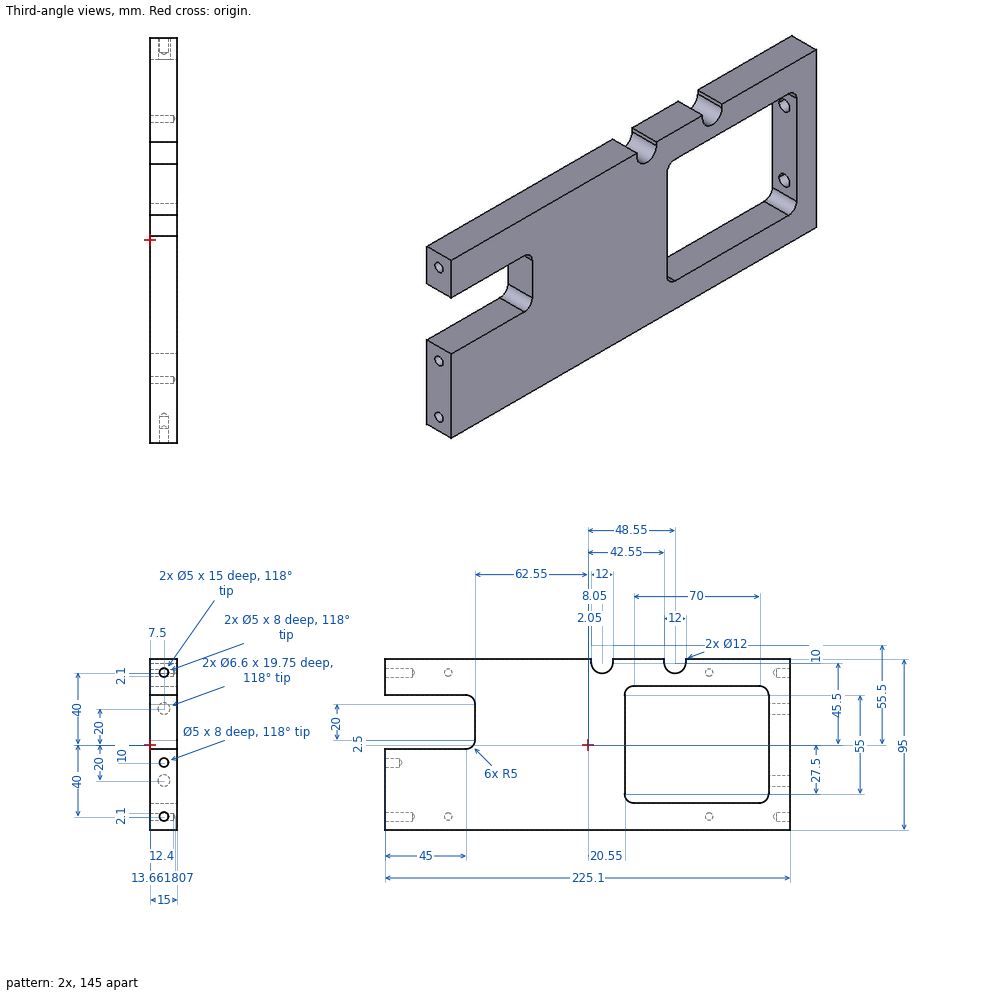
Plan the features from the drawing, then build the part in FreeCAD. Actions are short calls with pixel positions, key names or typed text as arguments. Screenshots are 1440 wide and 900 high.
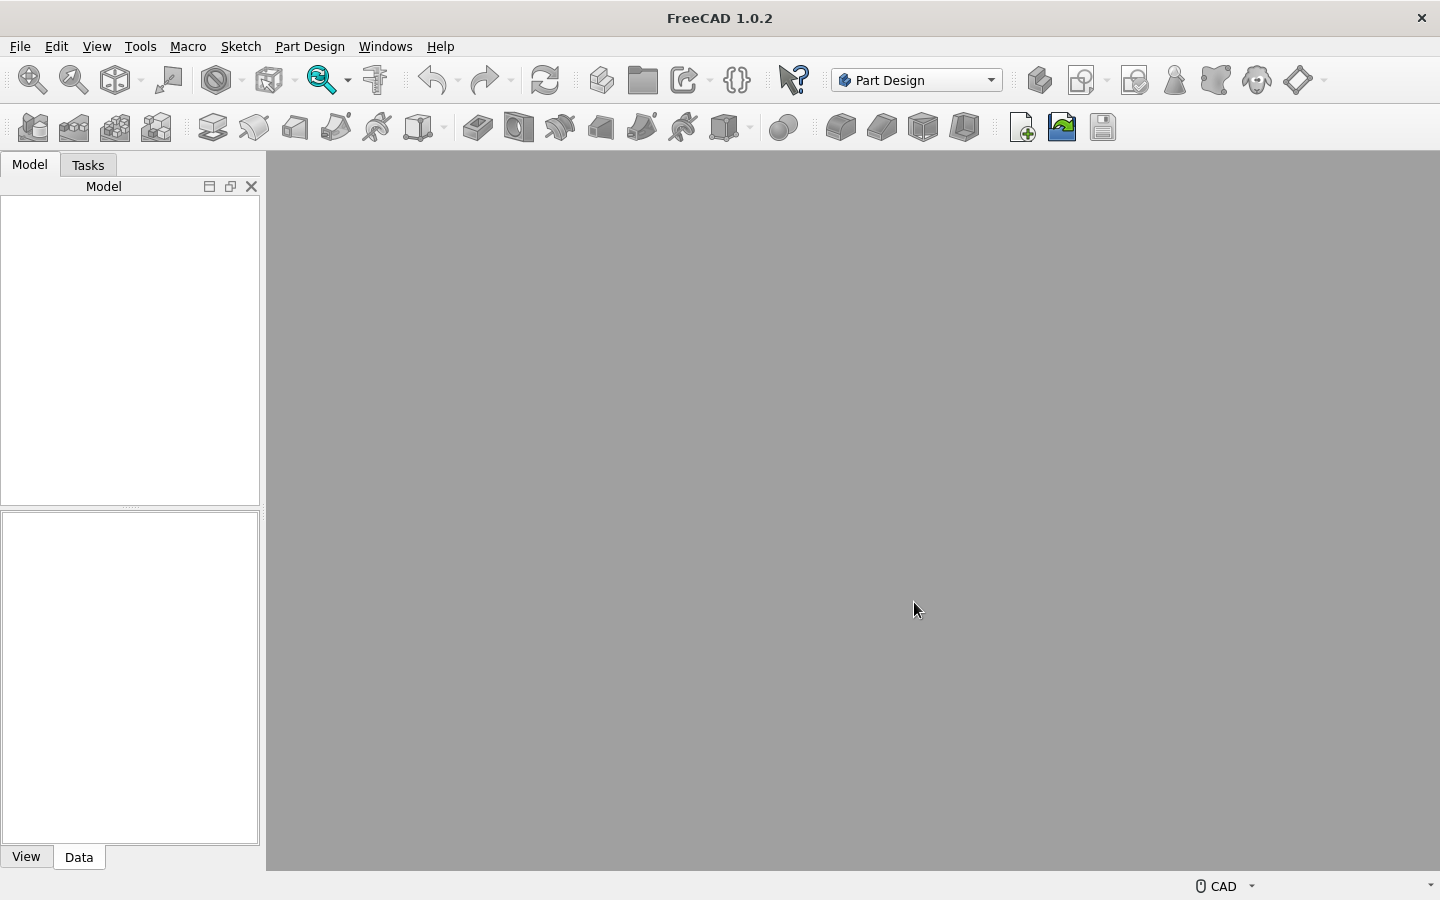
click(1021, 128)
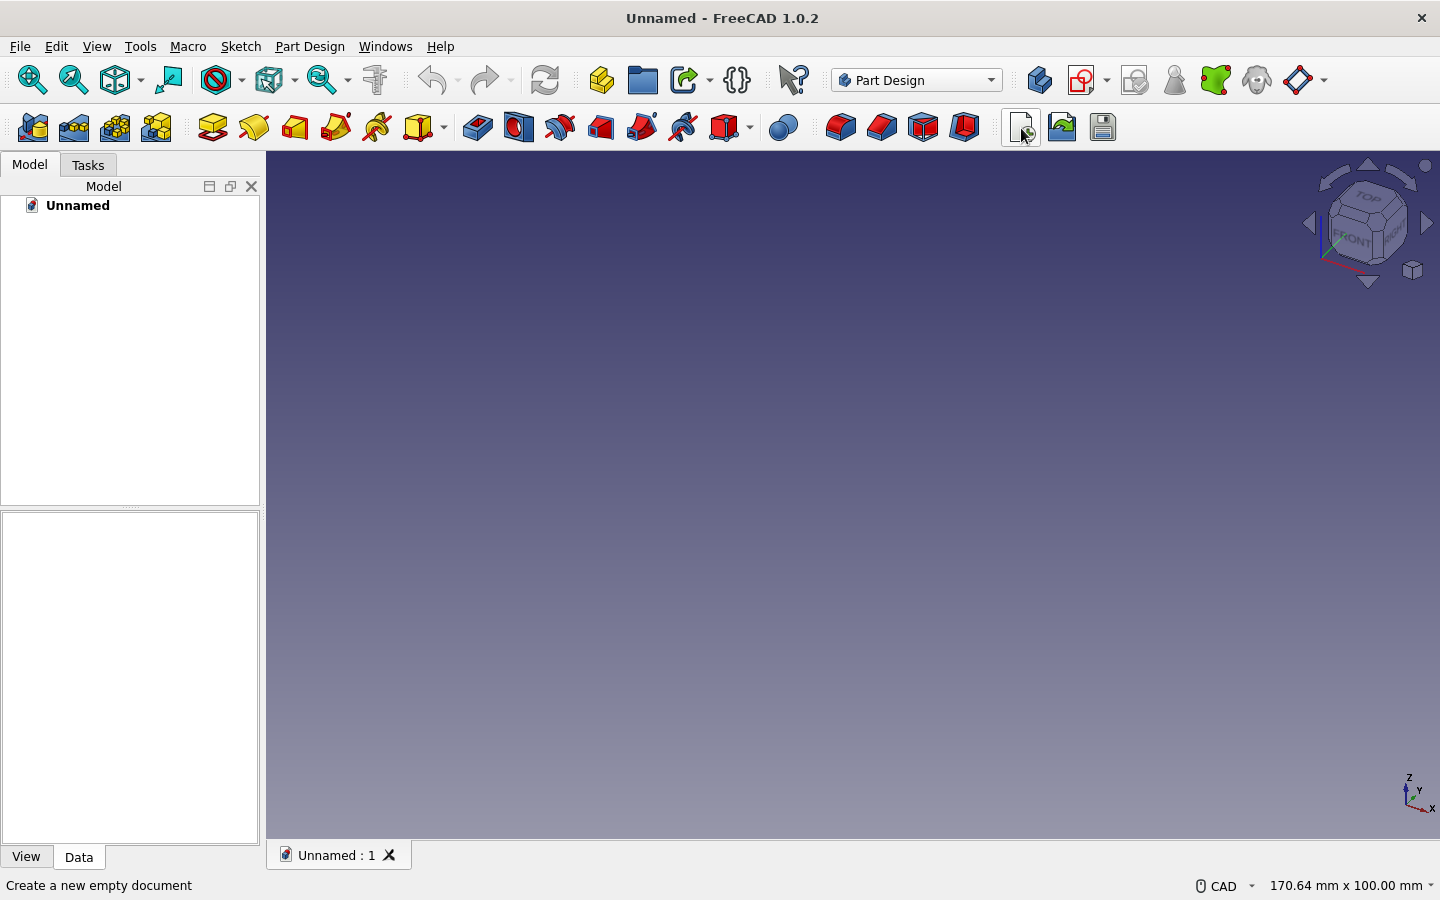
click(1080, 80)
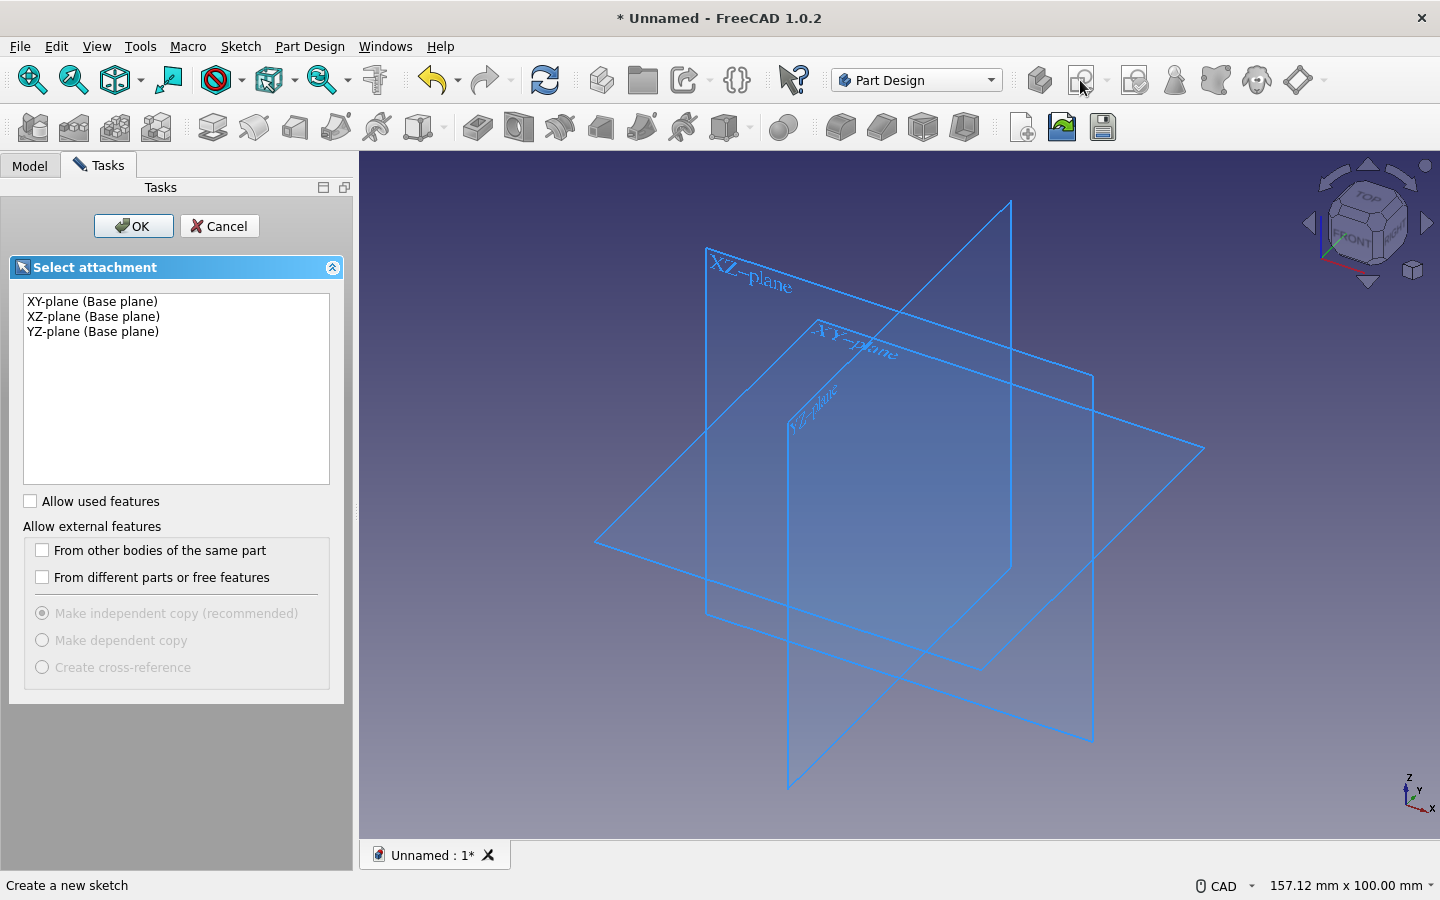
click(84, 332)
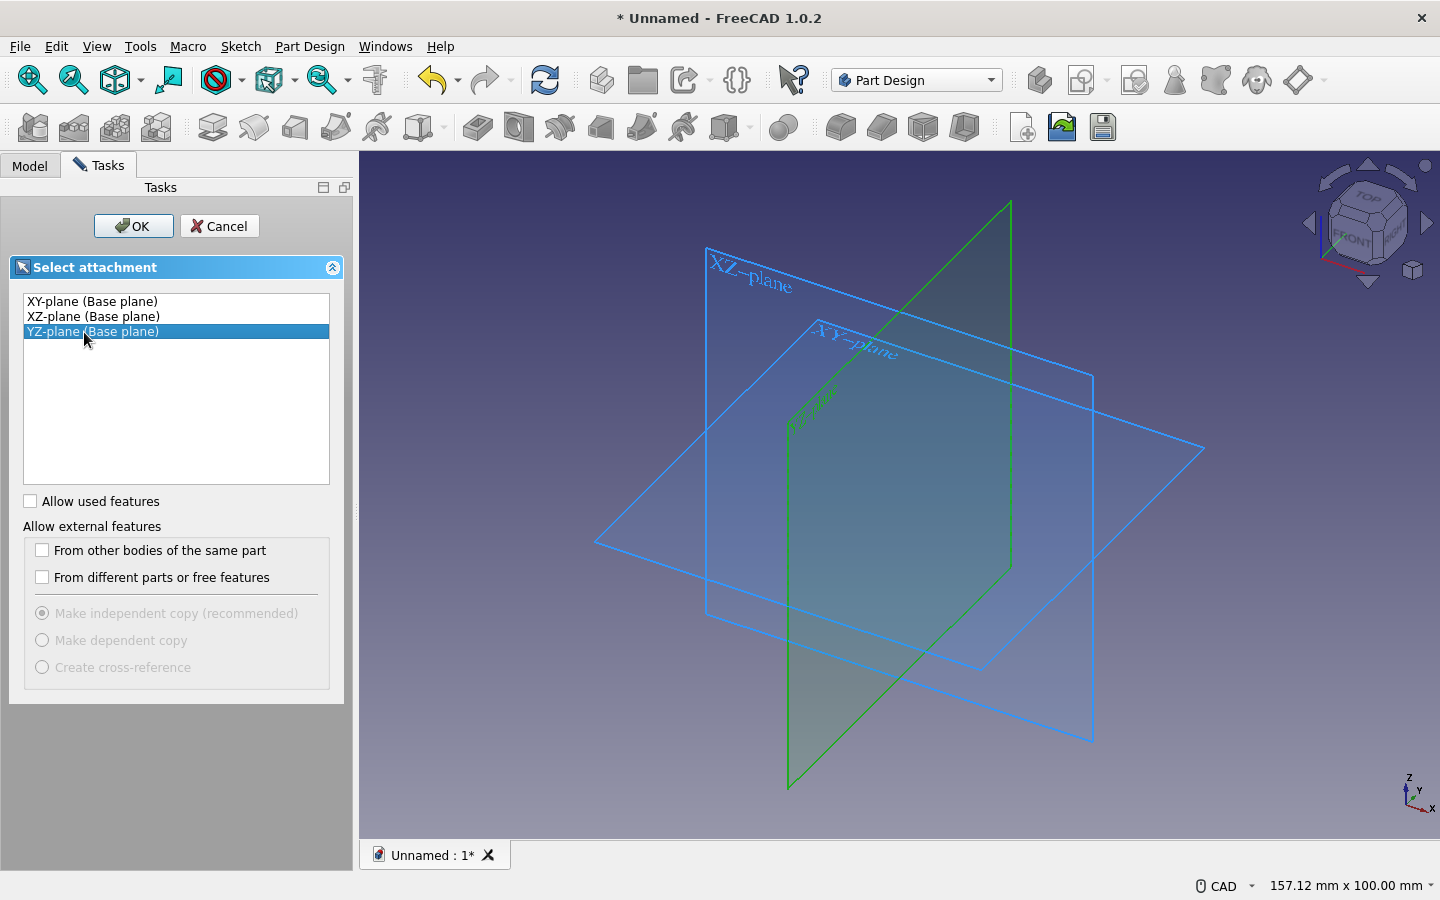
click(134, 226)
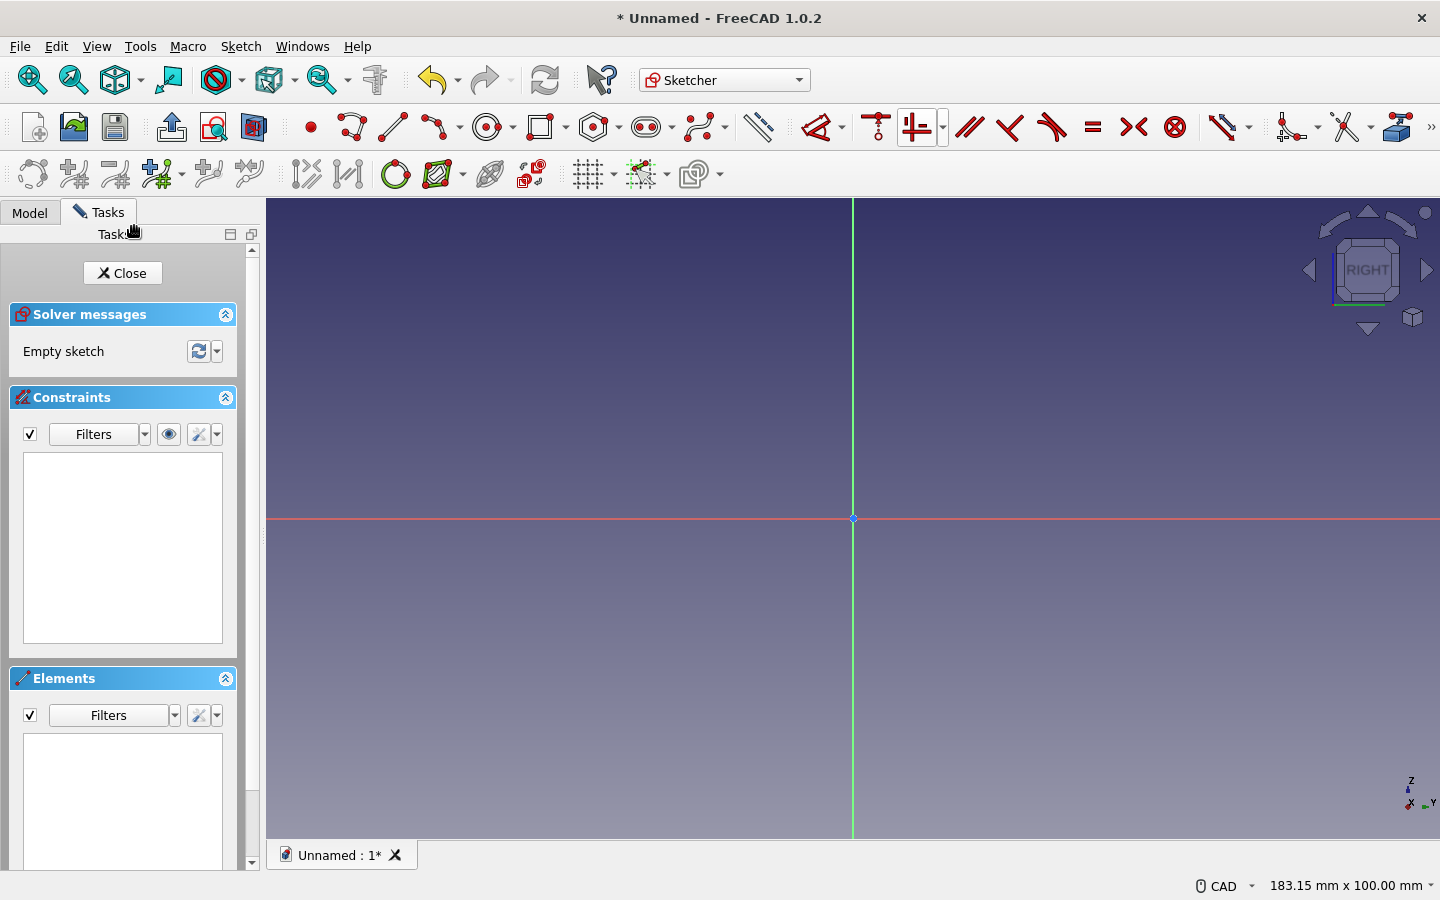
scroll(729, 519, down, 4)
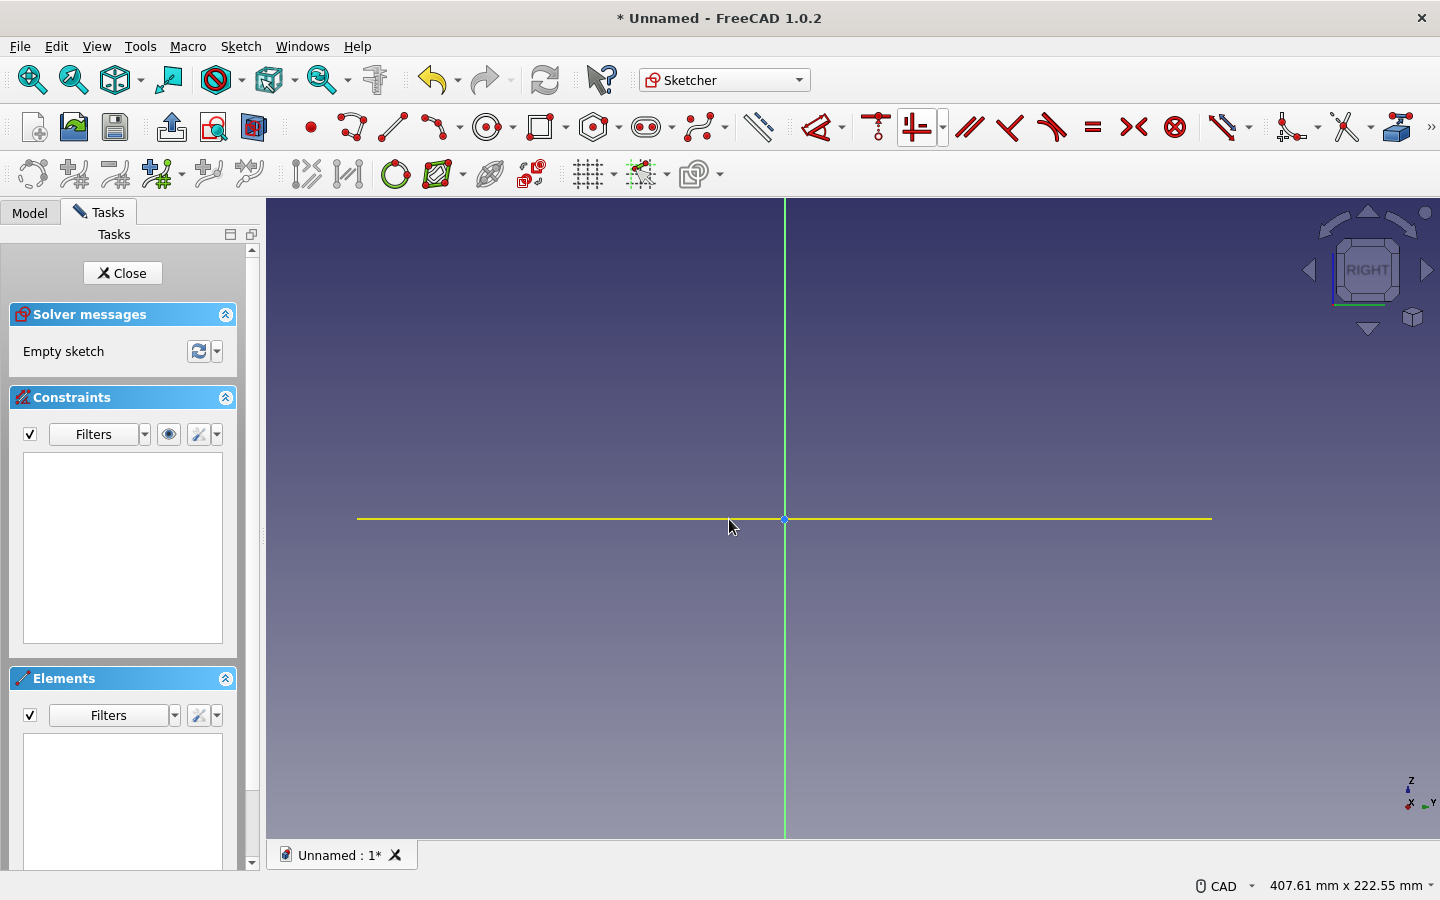
click(566, 128)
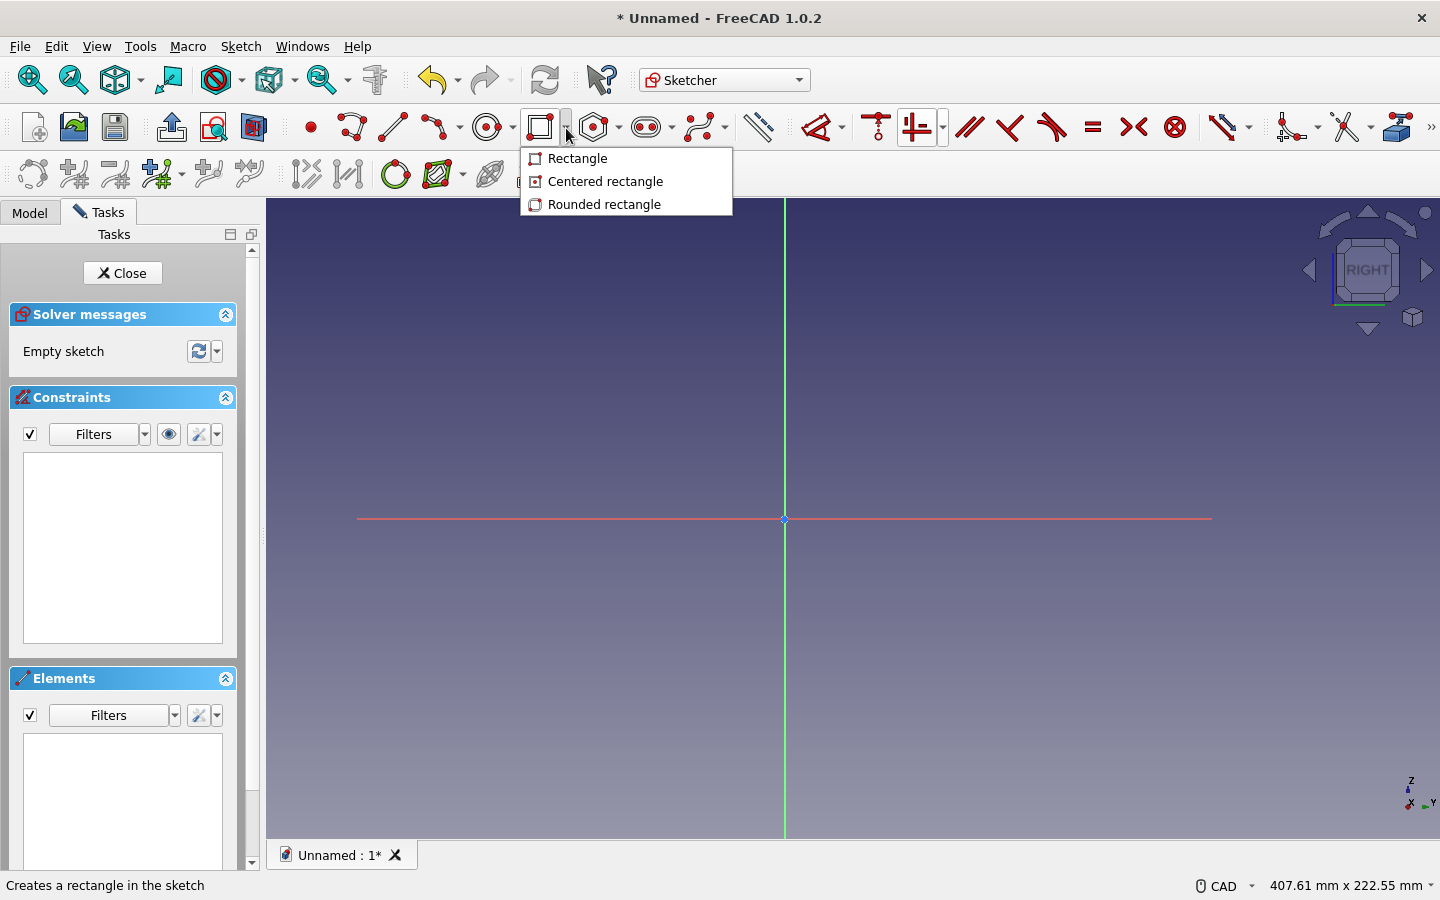
click(626, 182)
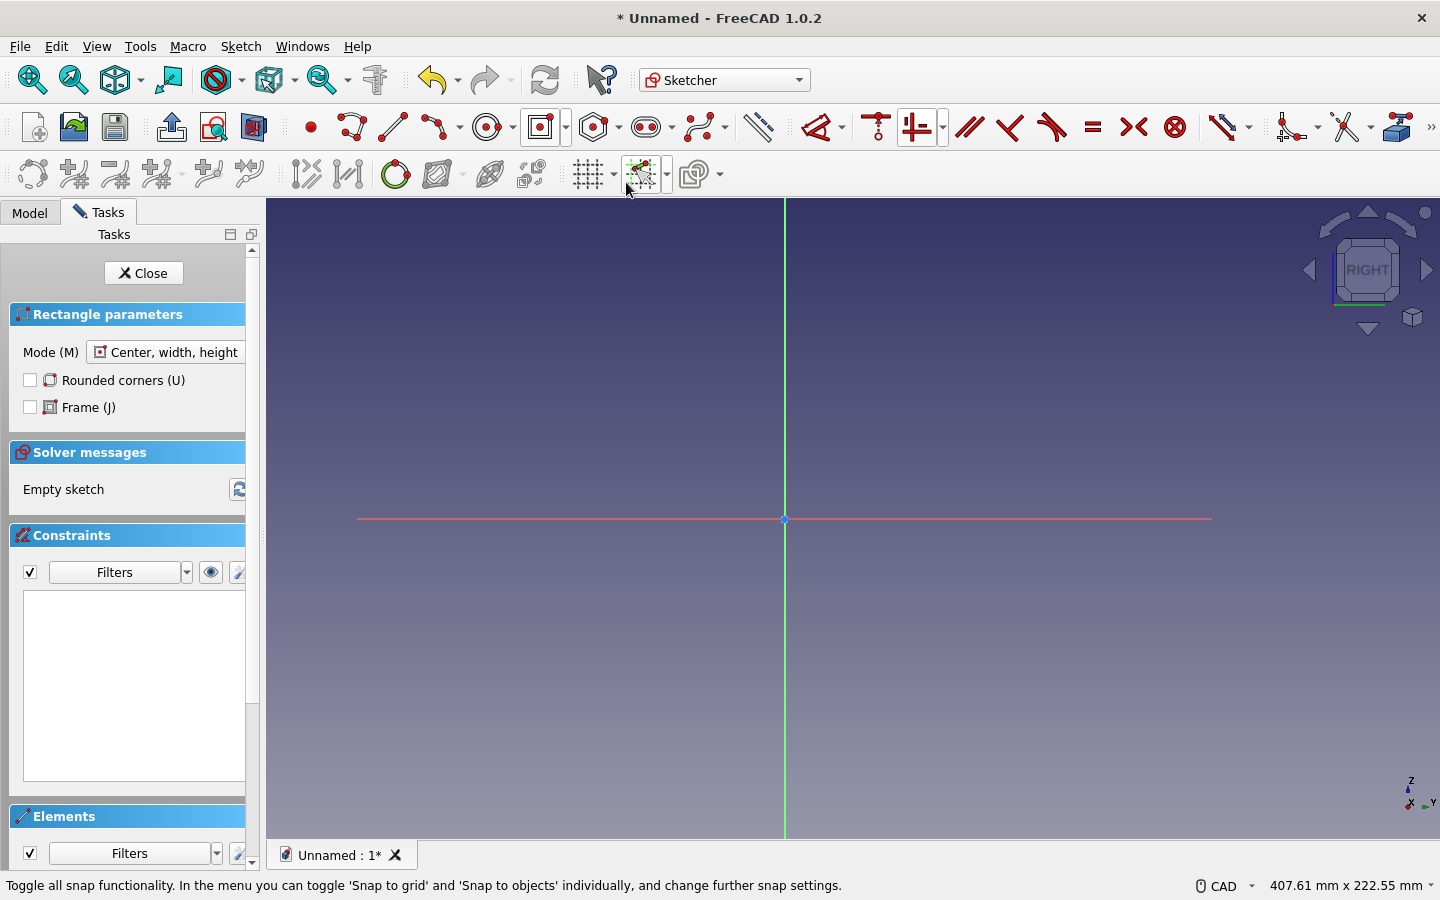
click(785, 519)
move(1109, 382)